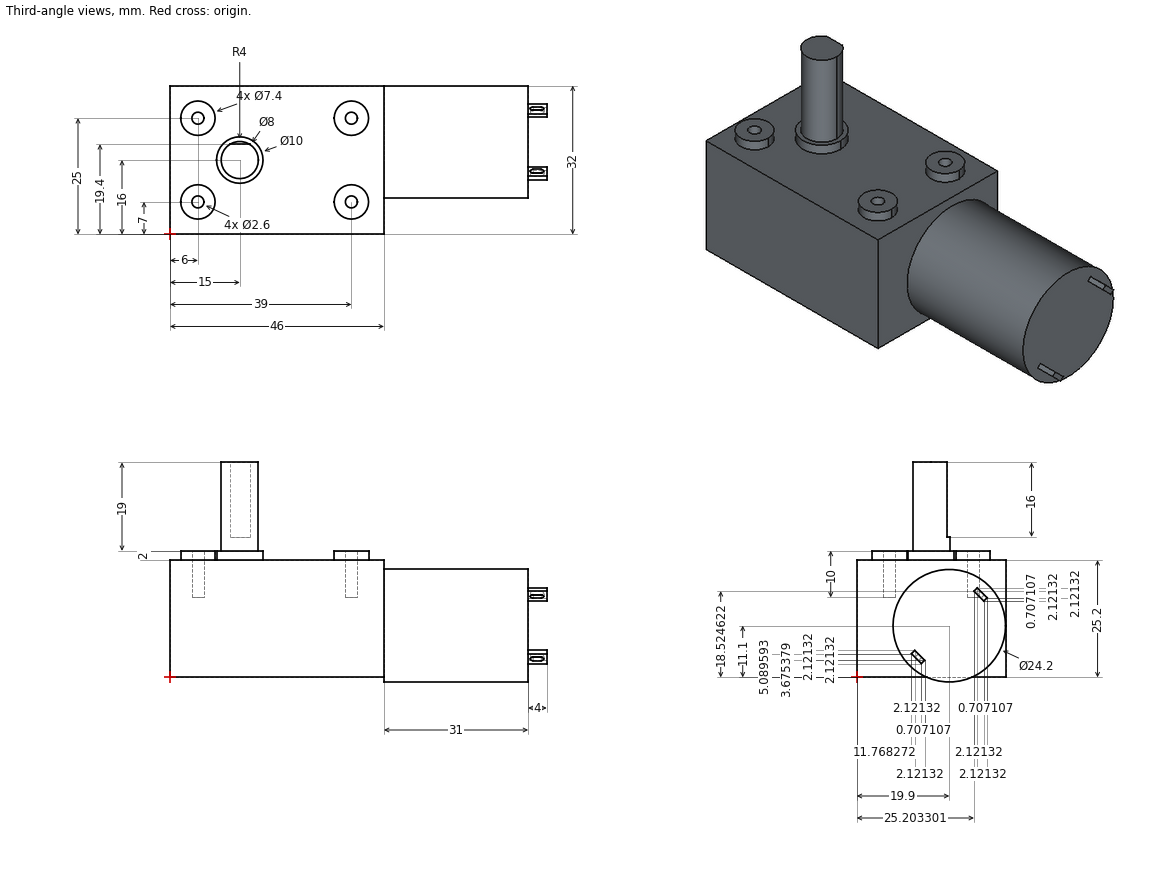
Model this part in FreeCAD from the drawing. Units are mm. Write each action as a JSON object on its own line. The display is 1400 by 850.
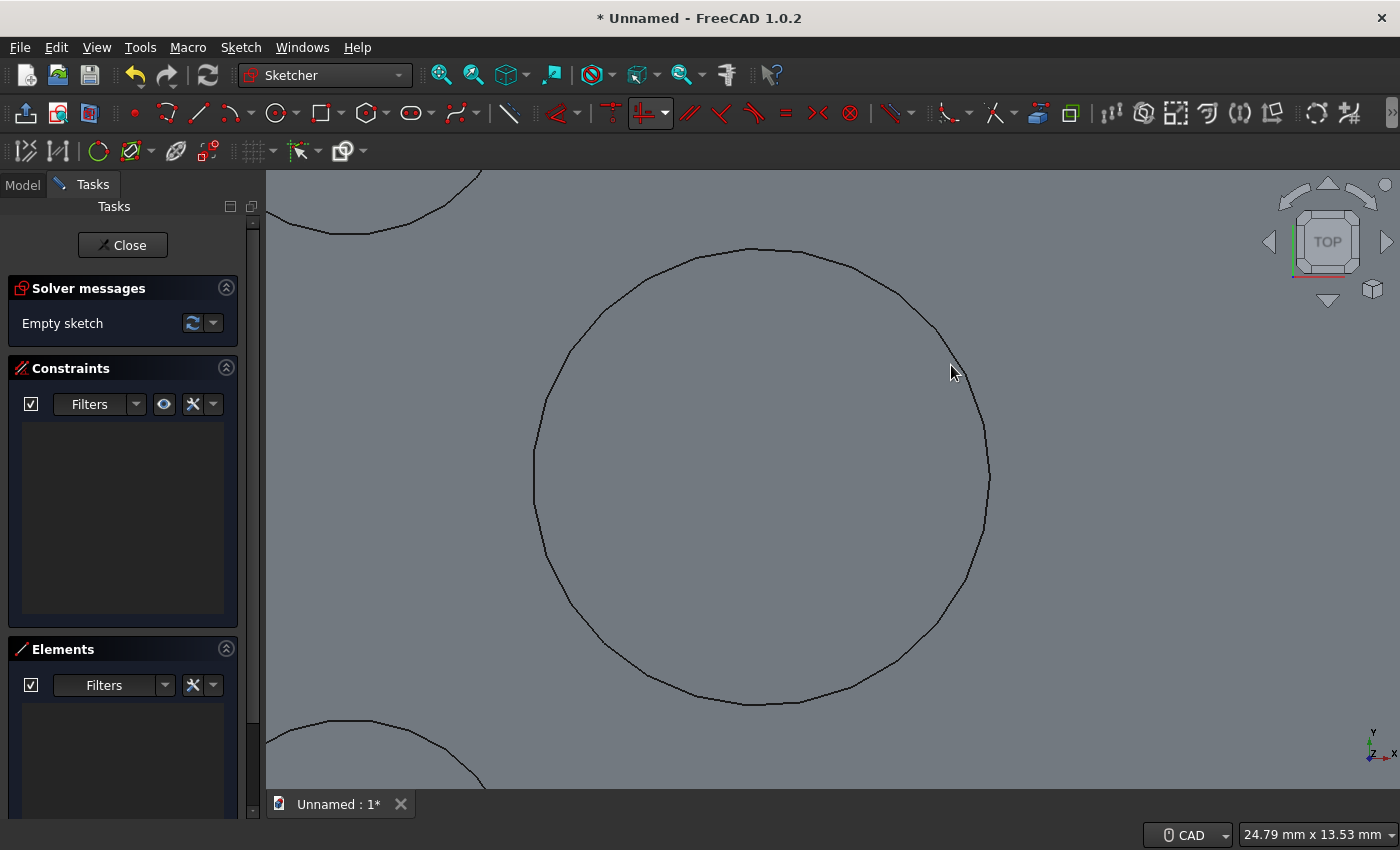
{"action": "left_click", "coordinate": [276, 114]}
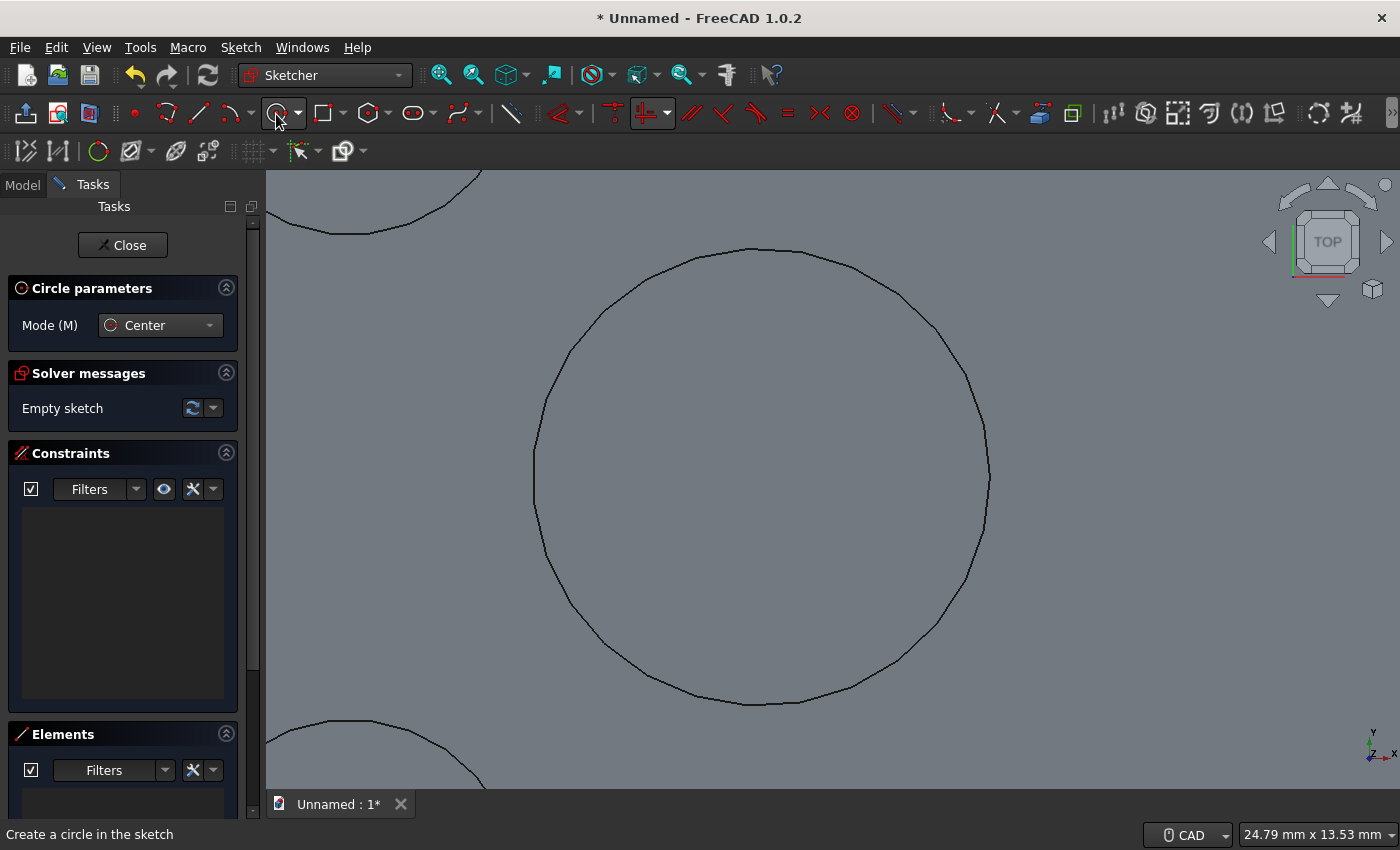
{"action": "left_click", "coordinate": [761, 477]}
{"action": "mouse_move", "coordinate": [891, 348]}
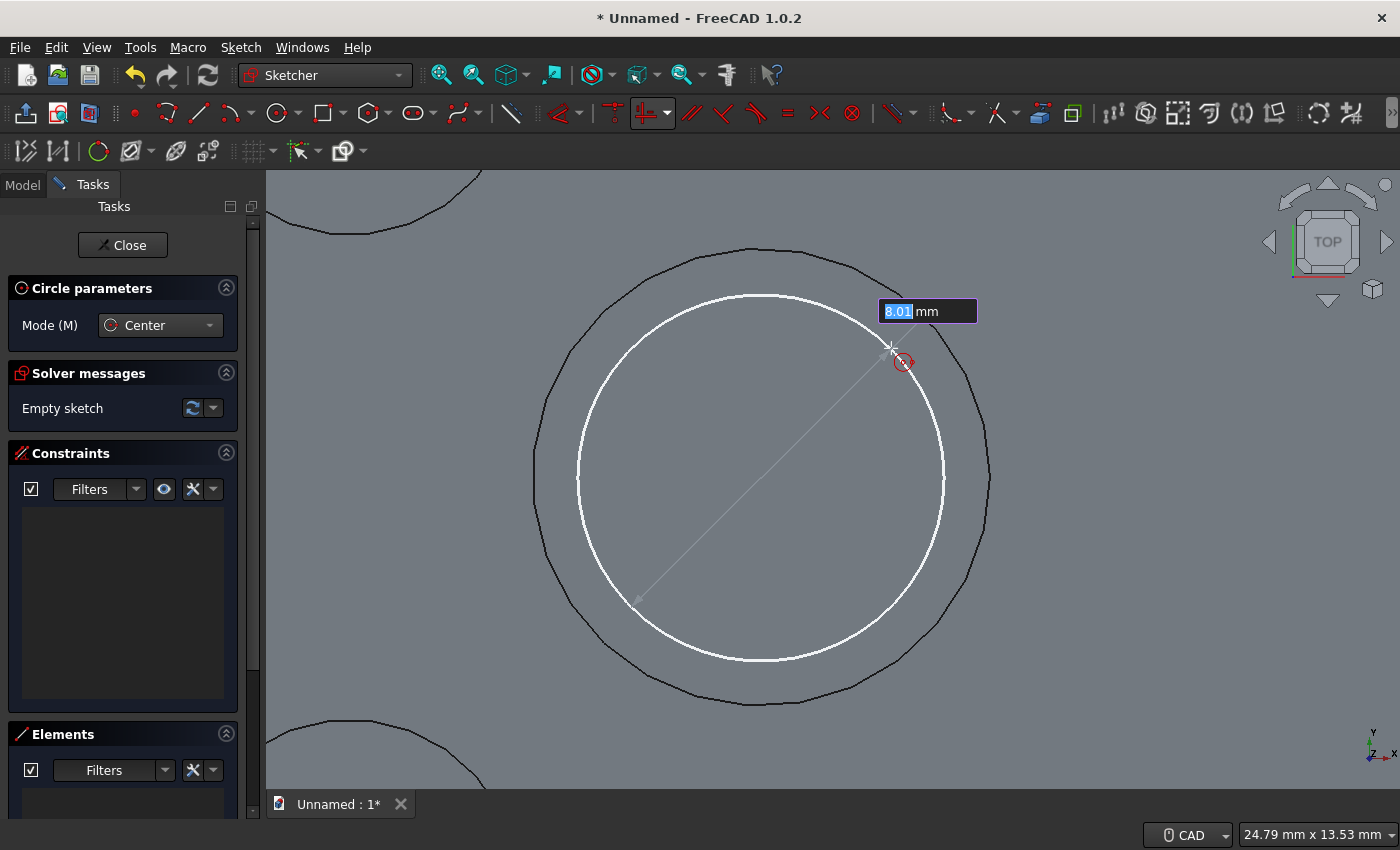
{"action": "type", "text": "8"}
{"action": "key", "text": "Return"}
{"action": "key", "text": "Escape"}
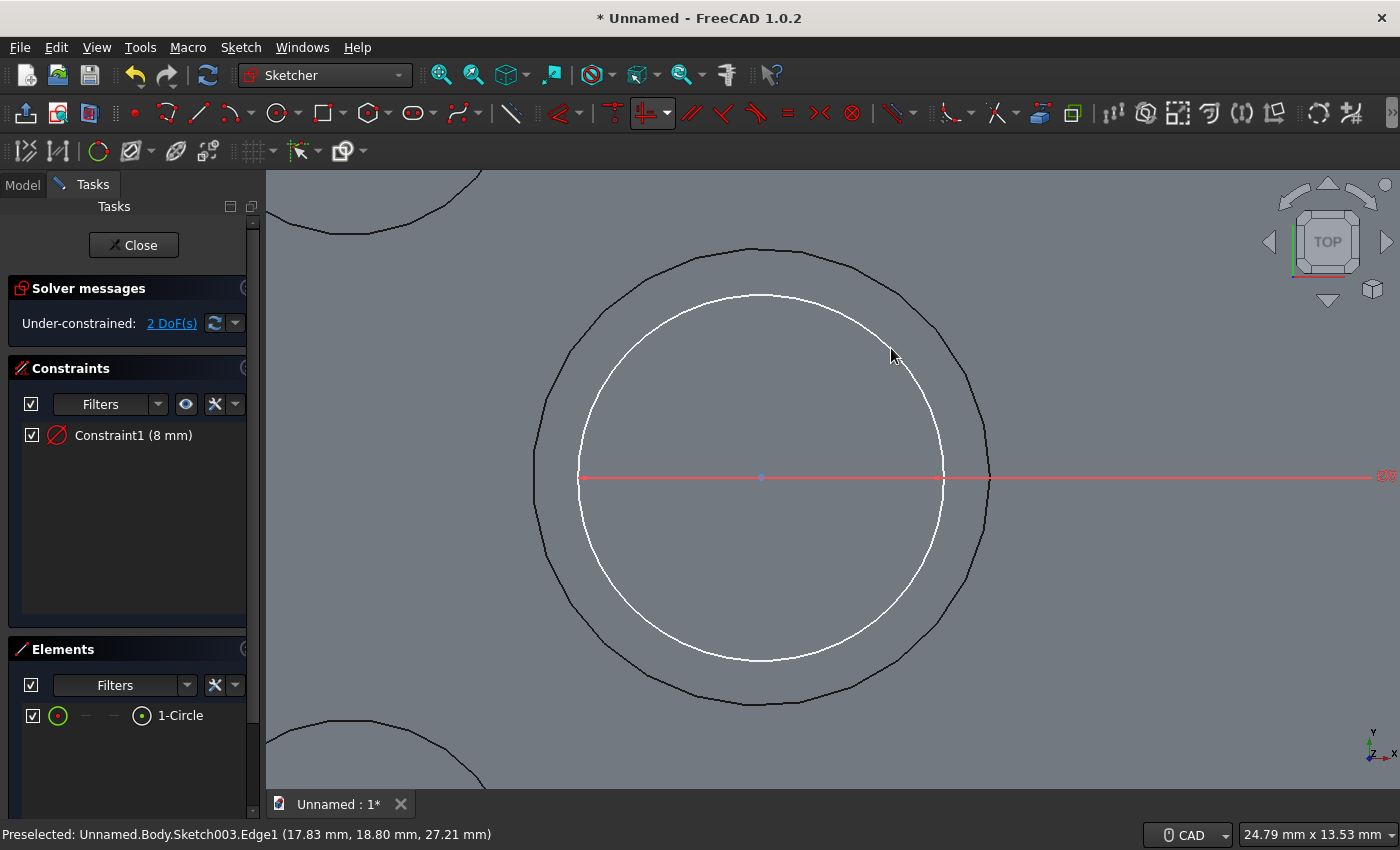
{"action": "key", "text": "d"}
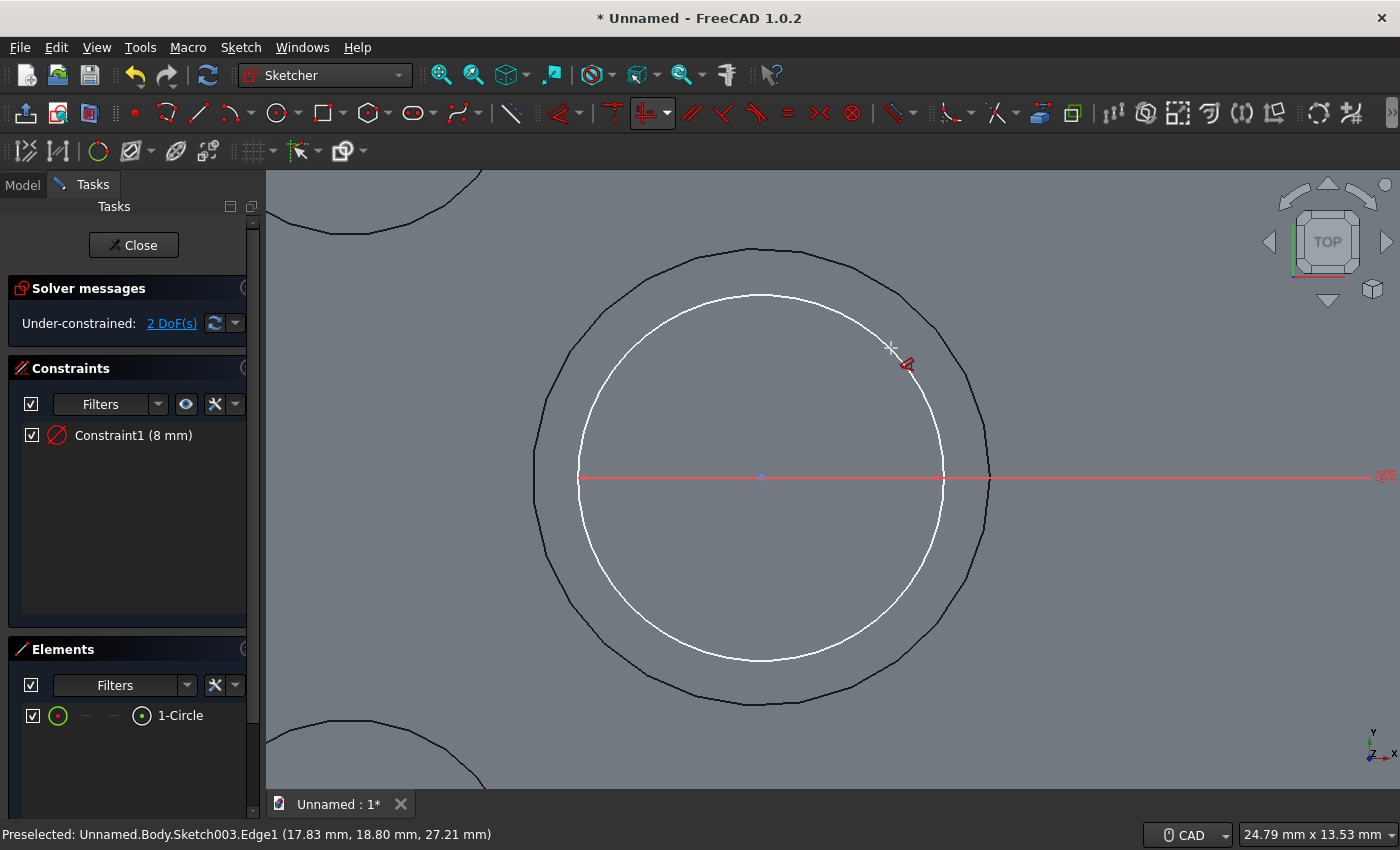
{"action": "left_click", "coordinate": [761, 478]}
{"action": "left_click", "coordinate": [527, 444]}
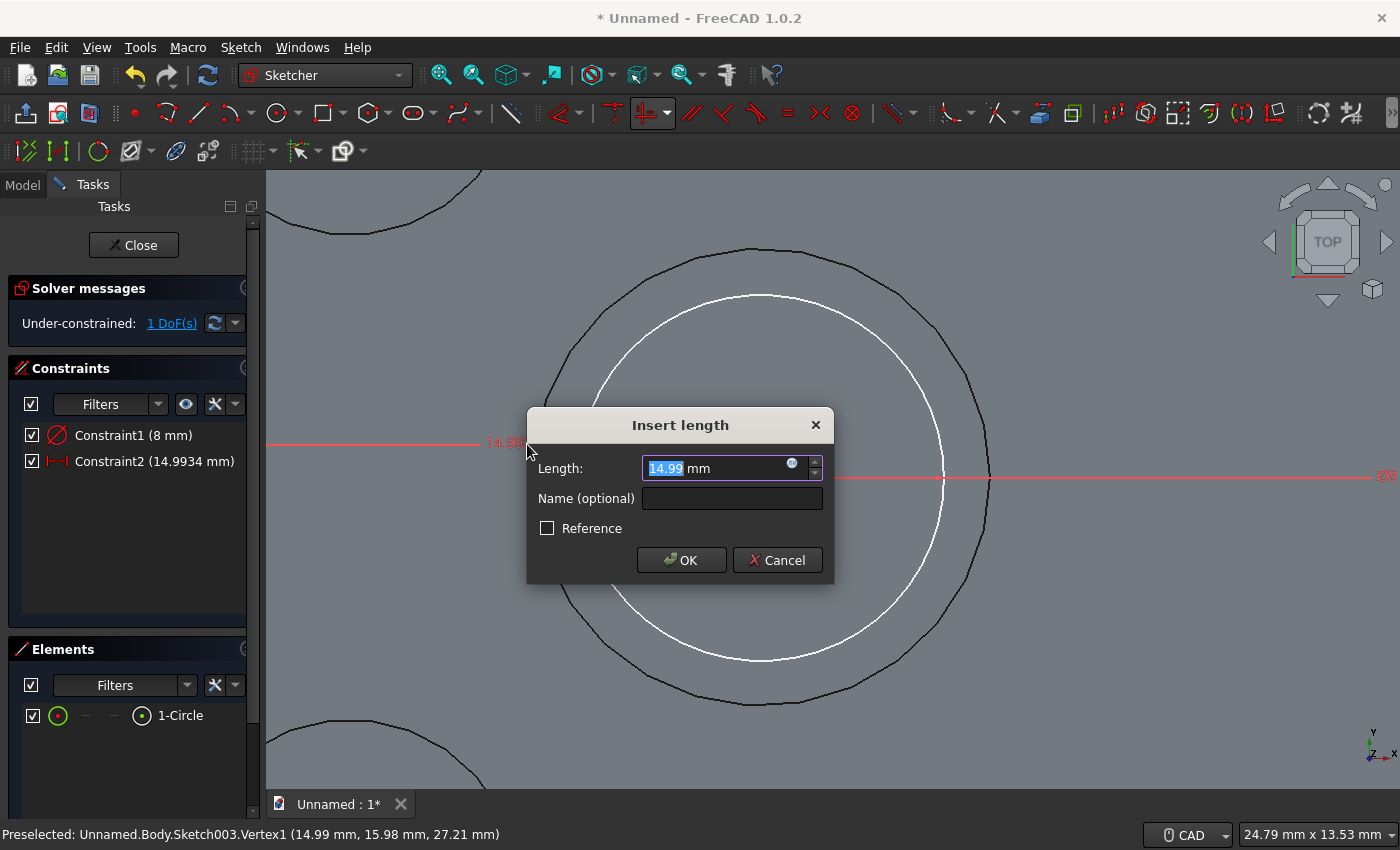
{"action": "type", "text": "15"}
{"action": "key", "text": "Return"}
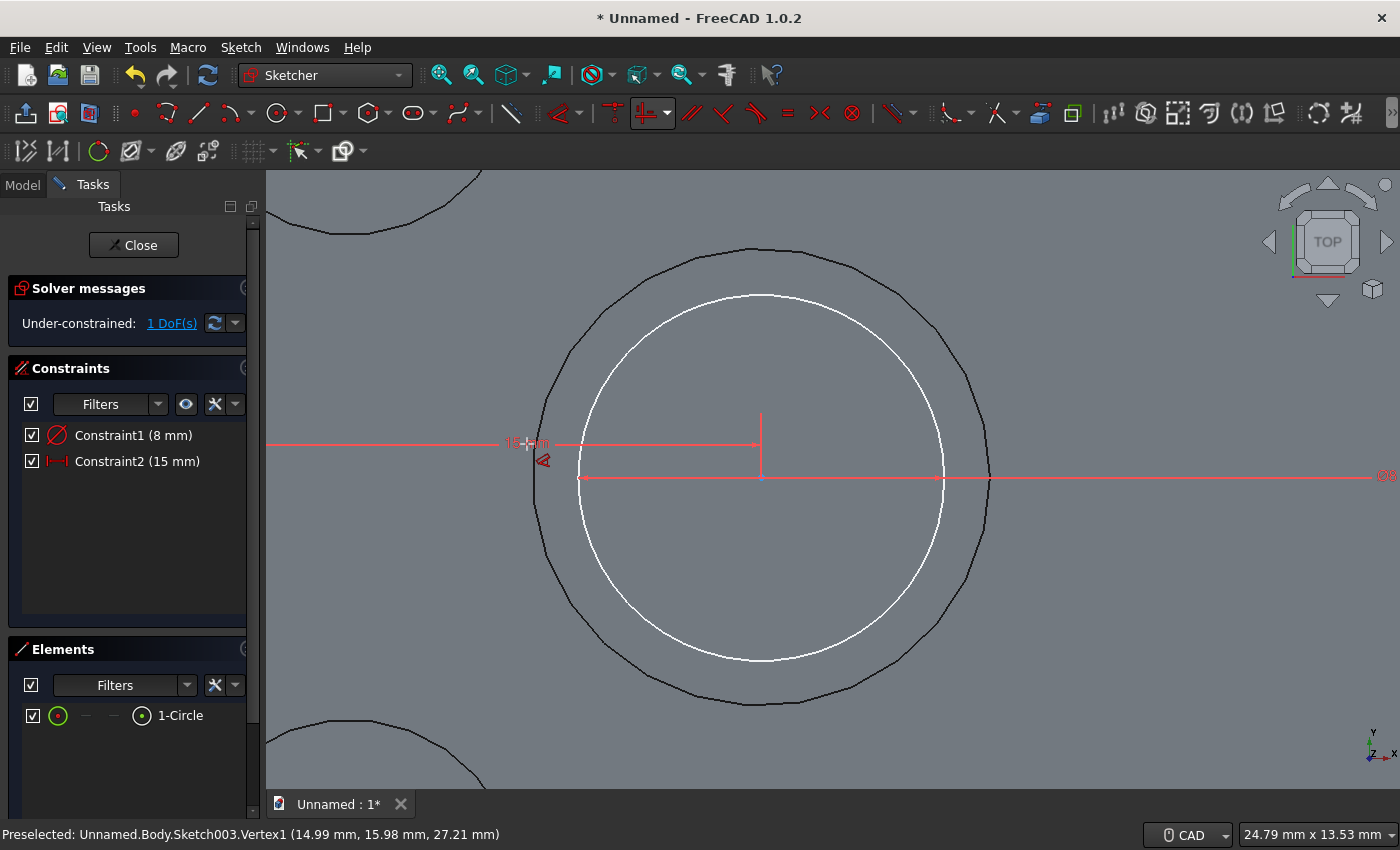
{"action": "left_click", "coordinate": [761, 478]}
{"action": "left_click", "coordinate": [795, 619]}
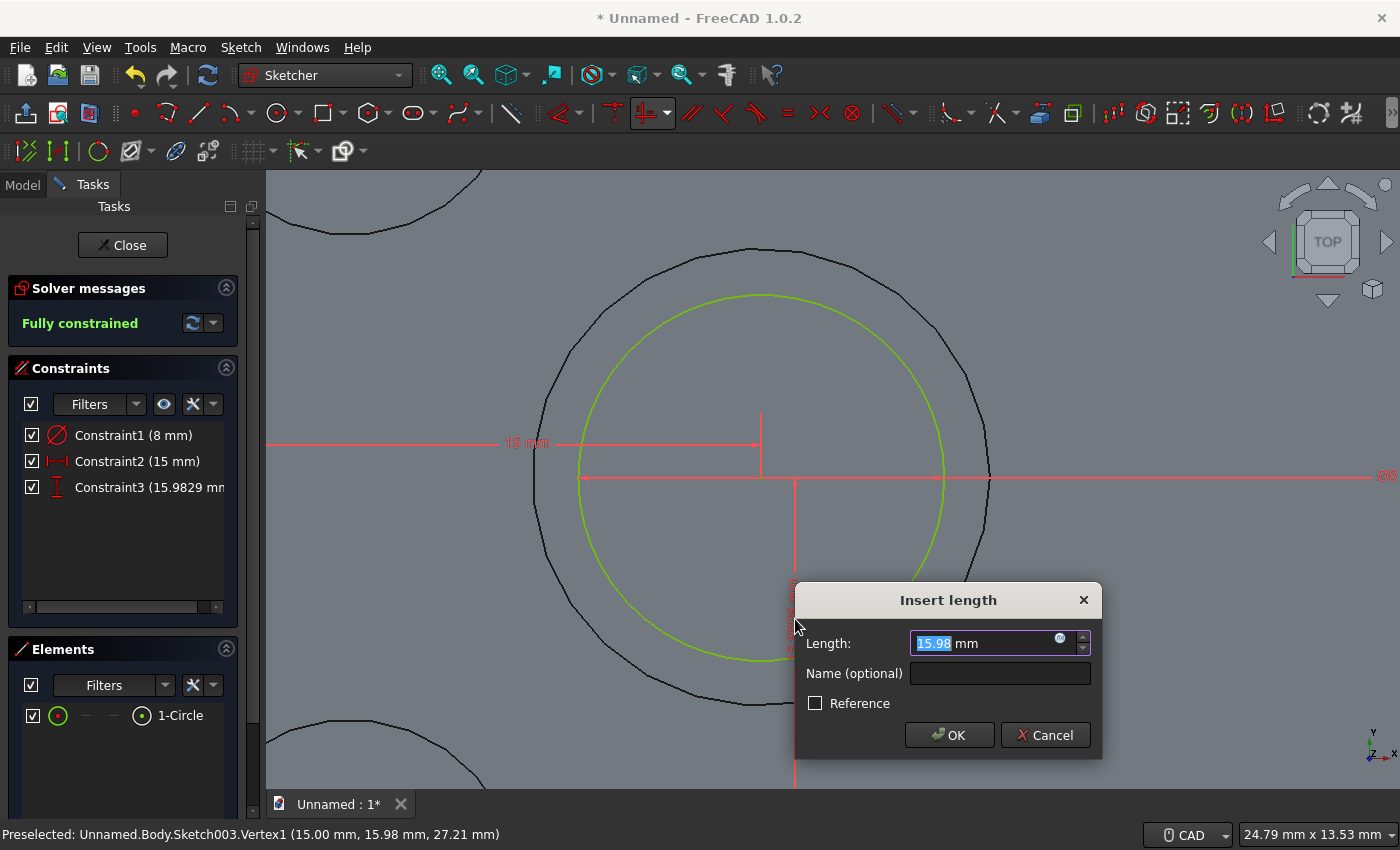
{"action": "type", "text": "16"}
{"action": "key", "text": "Return"}
{"action": "key", "text": "Escape"}